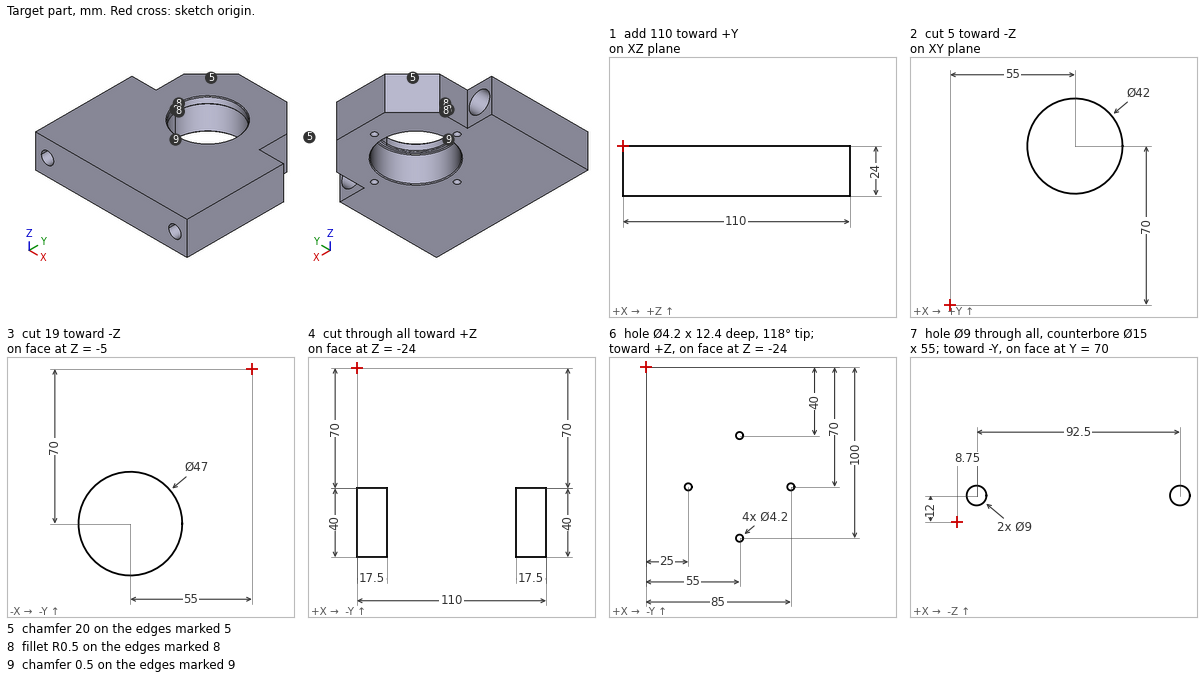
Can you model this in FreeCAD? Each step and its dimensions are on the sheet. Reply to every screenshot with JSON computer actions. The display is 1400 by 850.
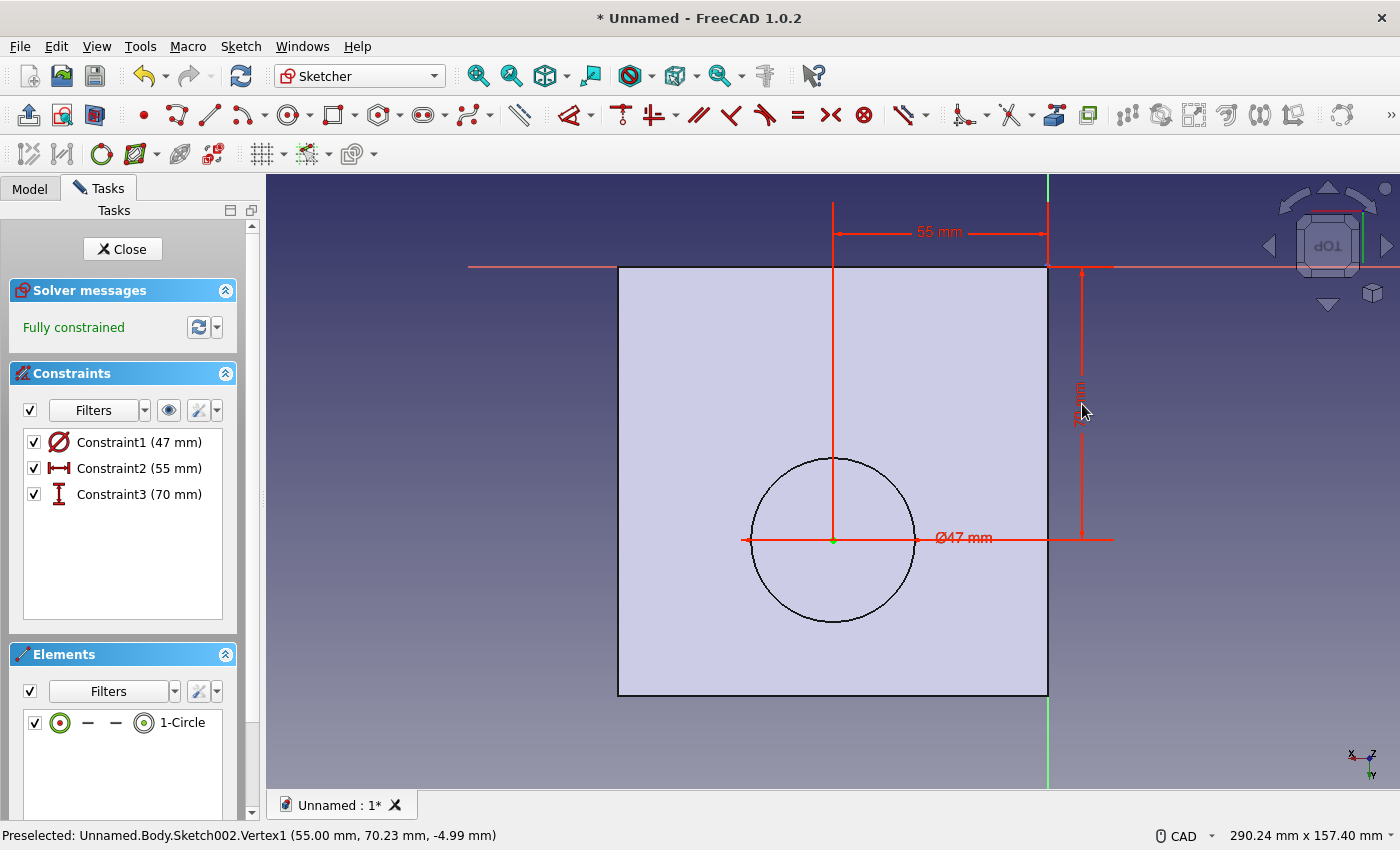
{"action": "left_click", "coordinate": [123, 249]}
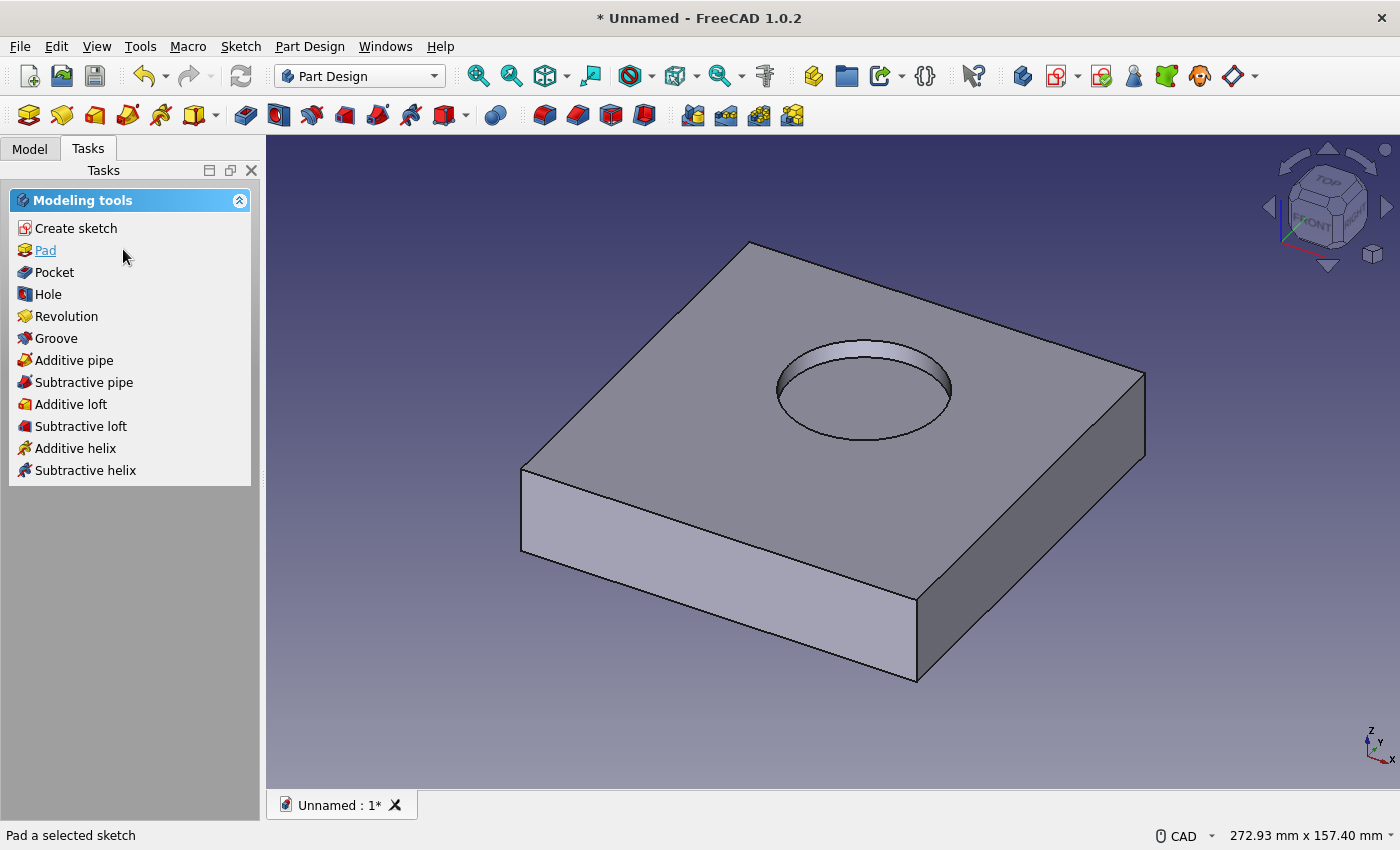
{"action": "left_click", "coordinate": [246, 116]}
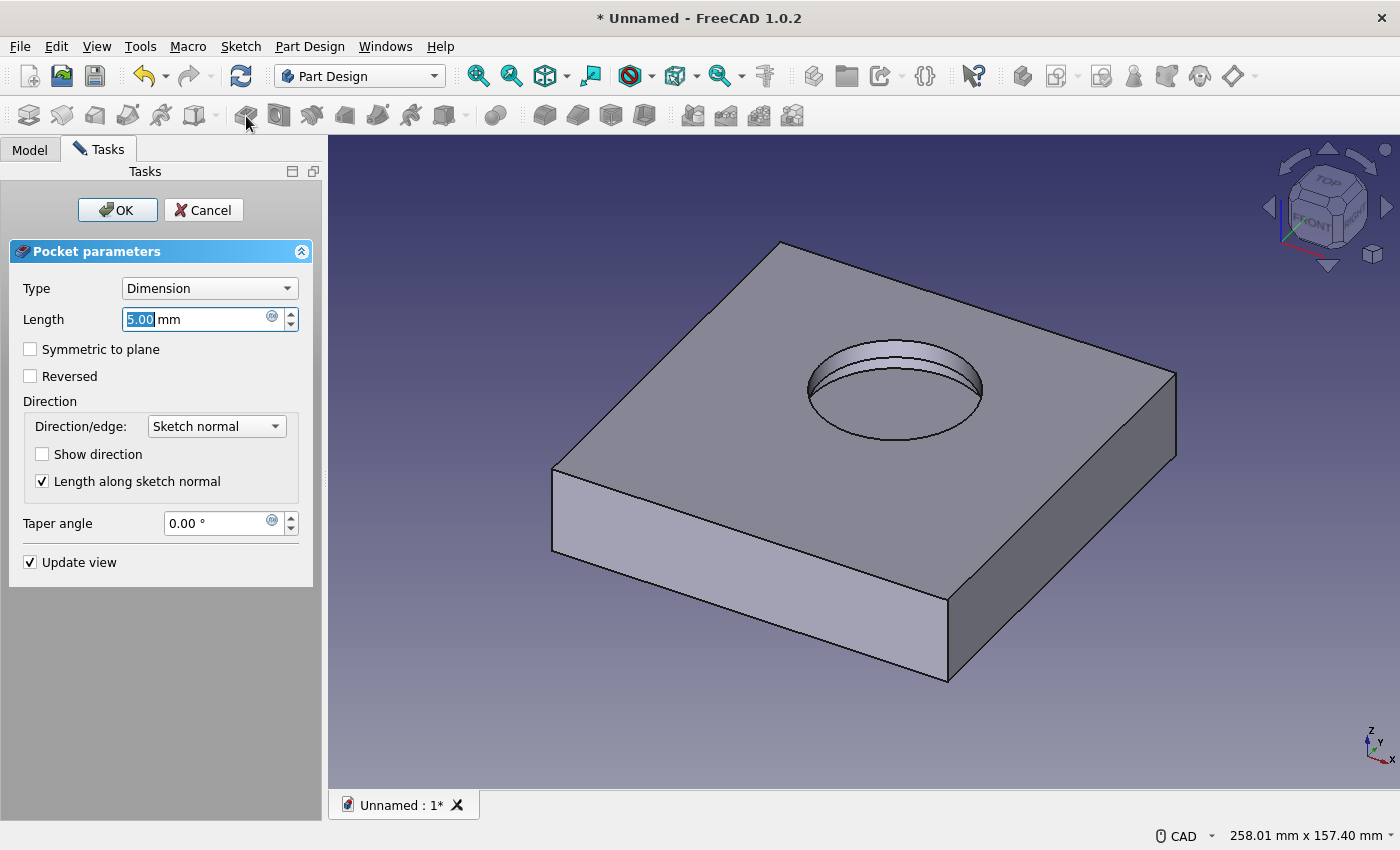
{"action": "type", "text": "19"}
{"action": "key", "text": "Tab"}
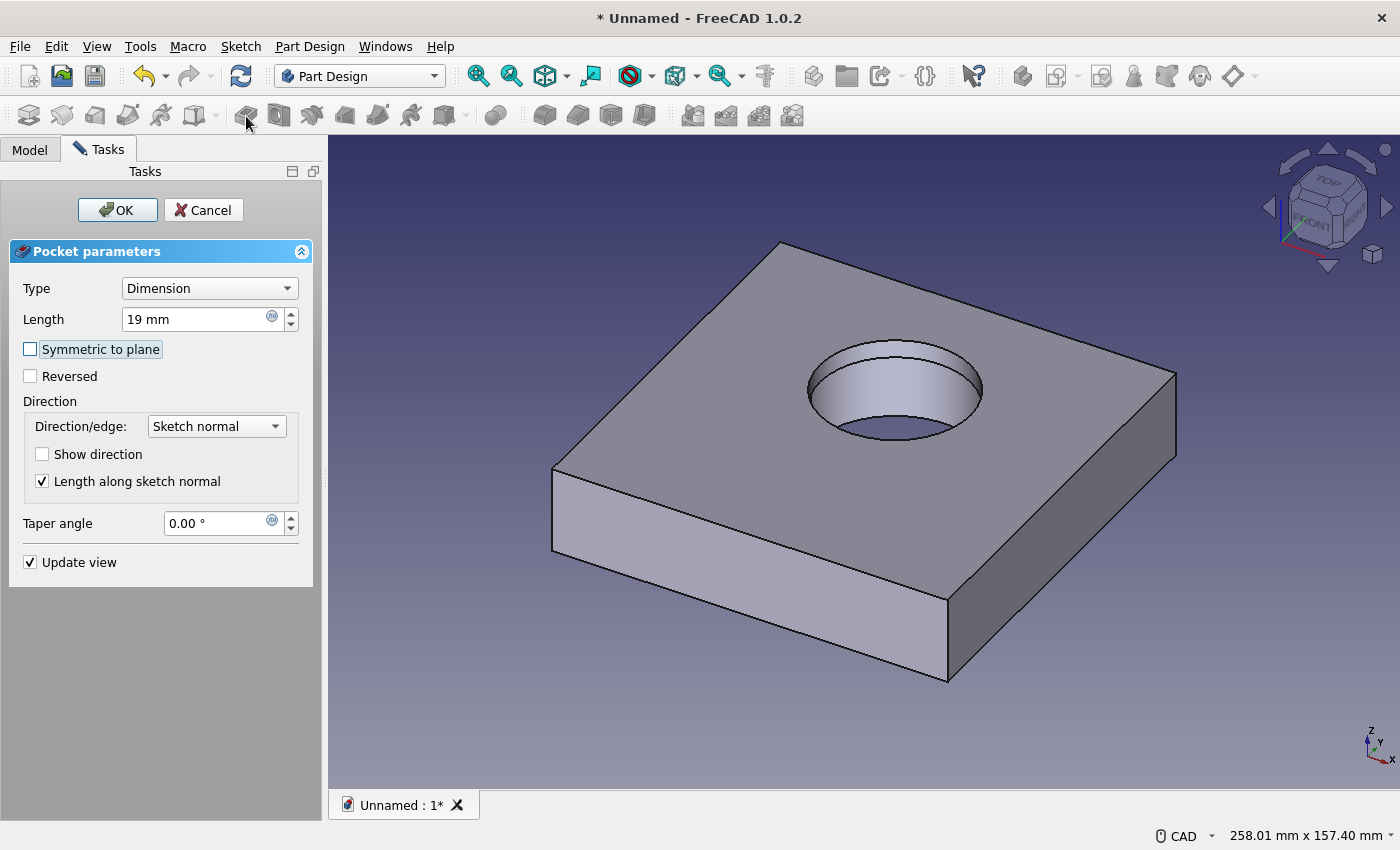
{"action": "left_click", "coordinate": [118, 210]}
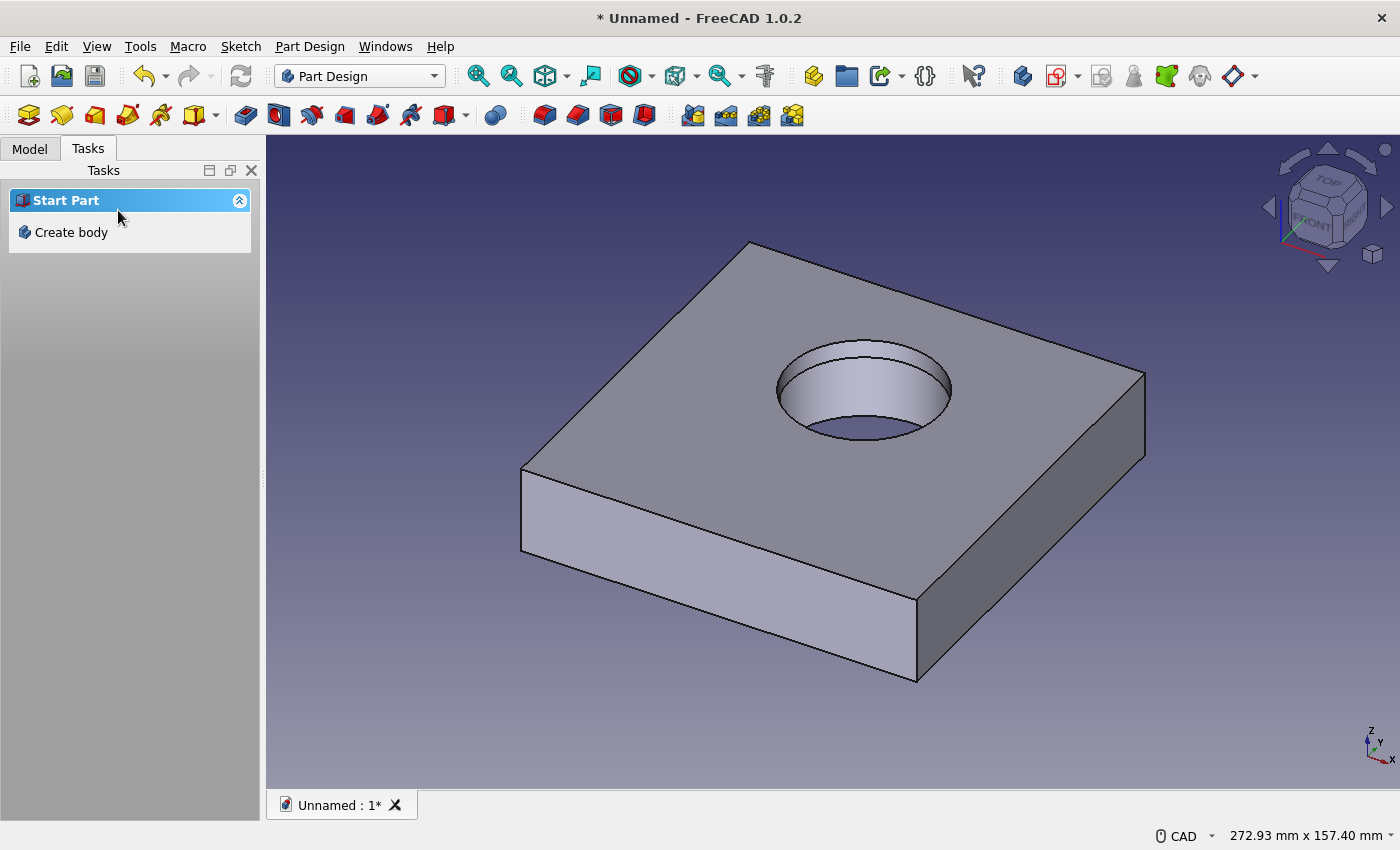
{"action": "key", "text": "5"}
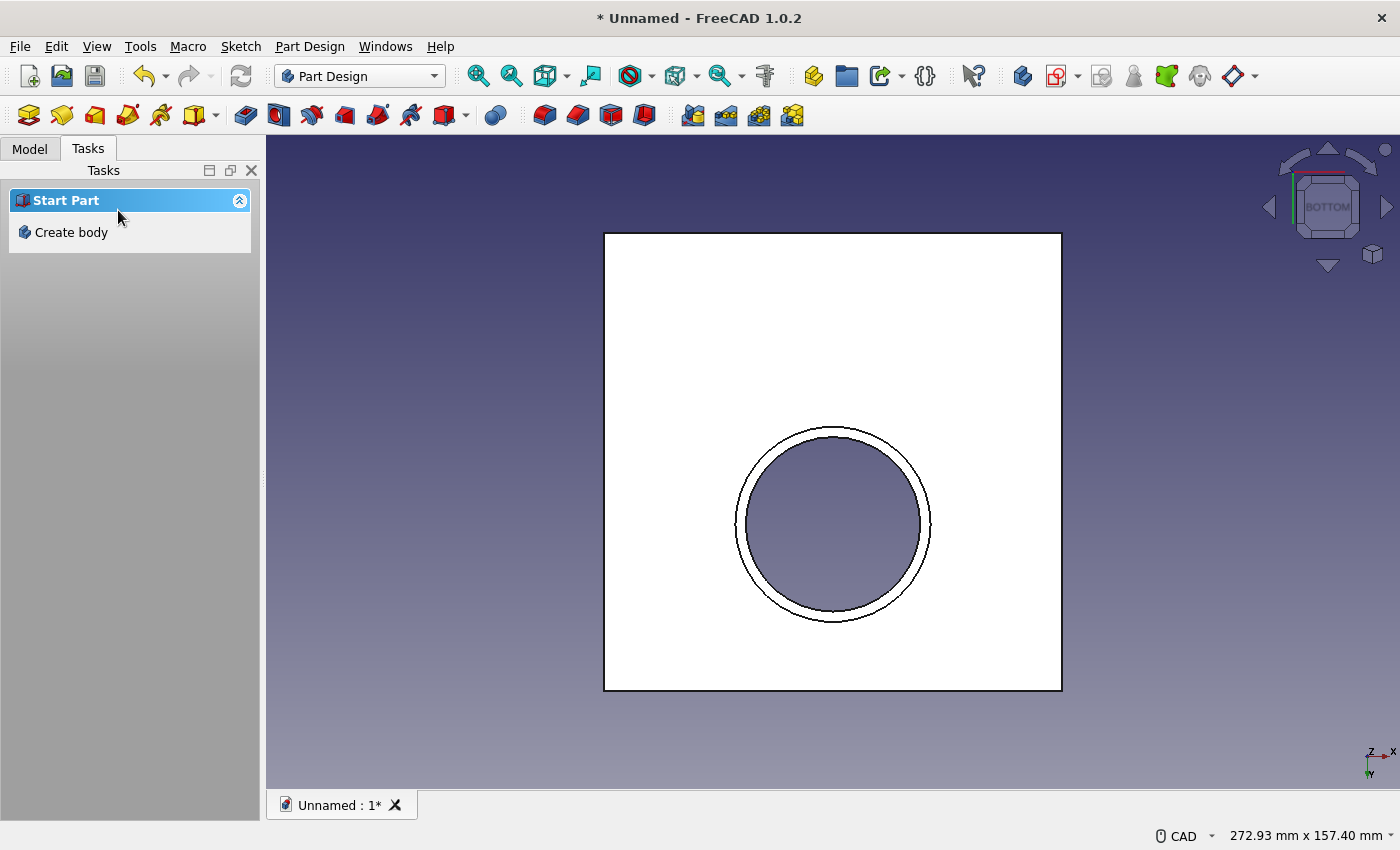
{"action": "left_click", "coordinate": [964, 330]}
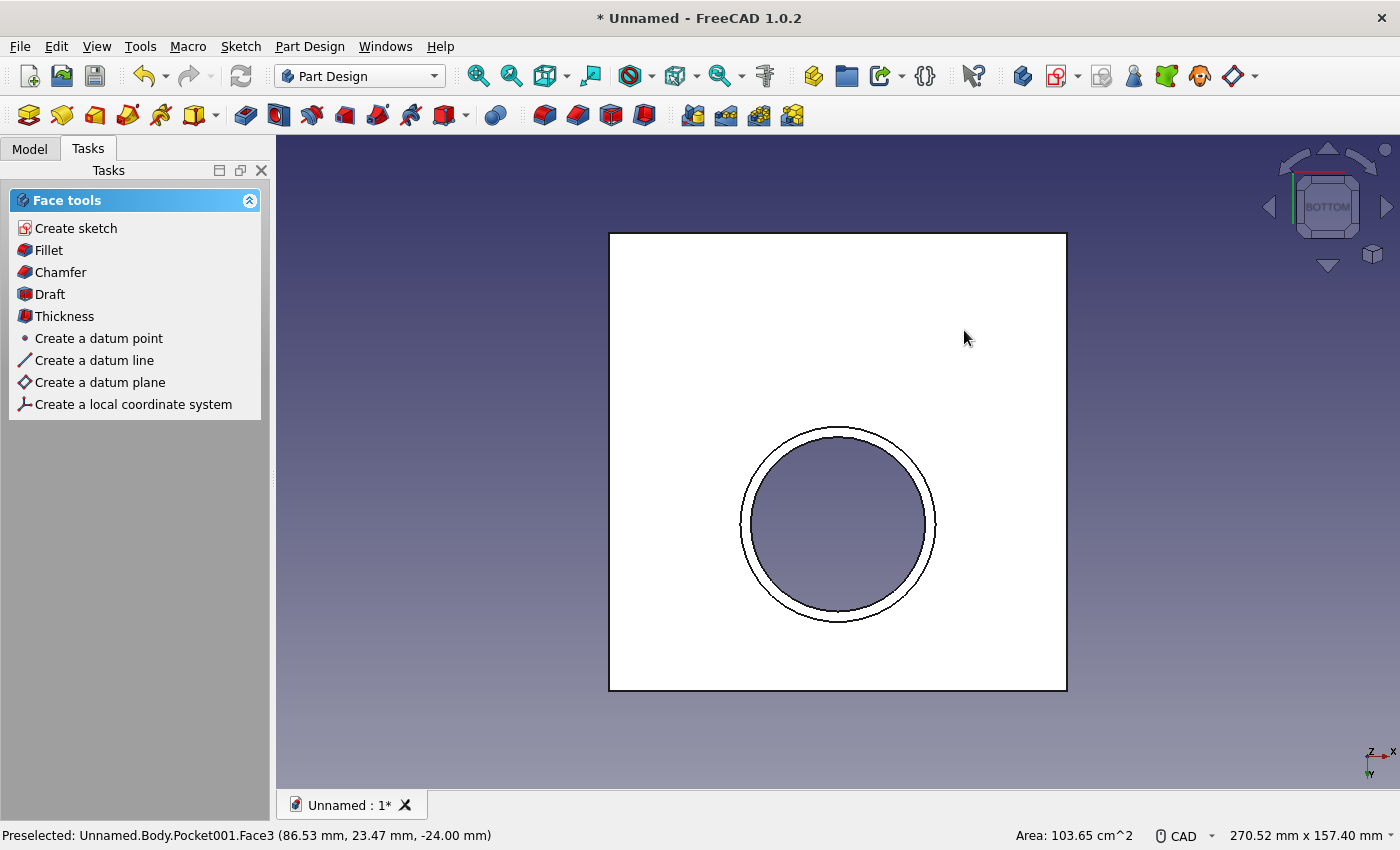
{"action": "left_click", "coordinate": [1056, 76]}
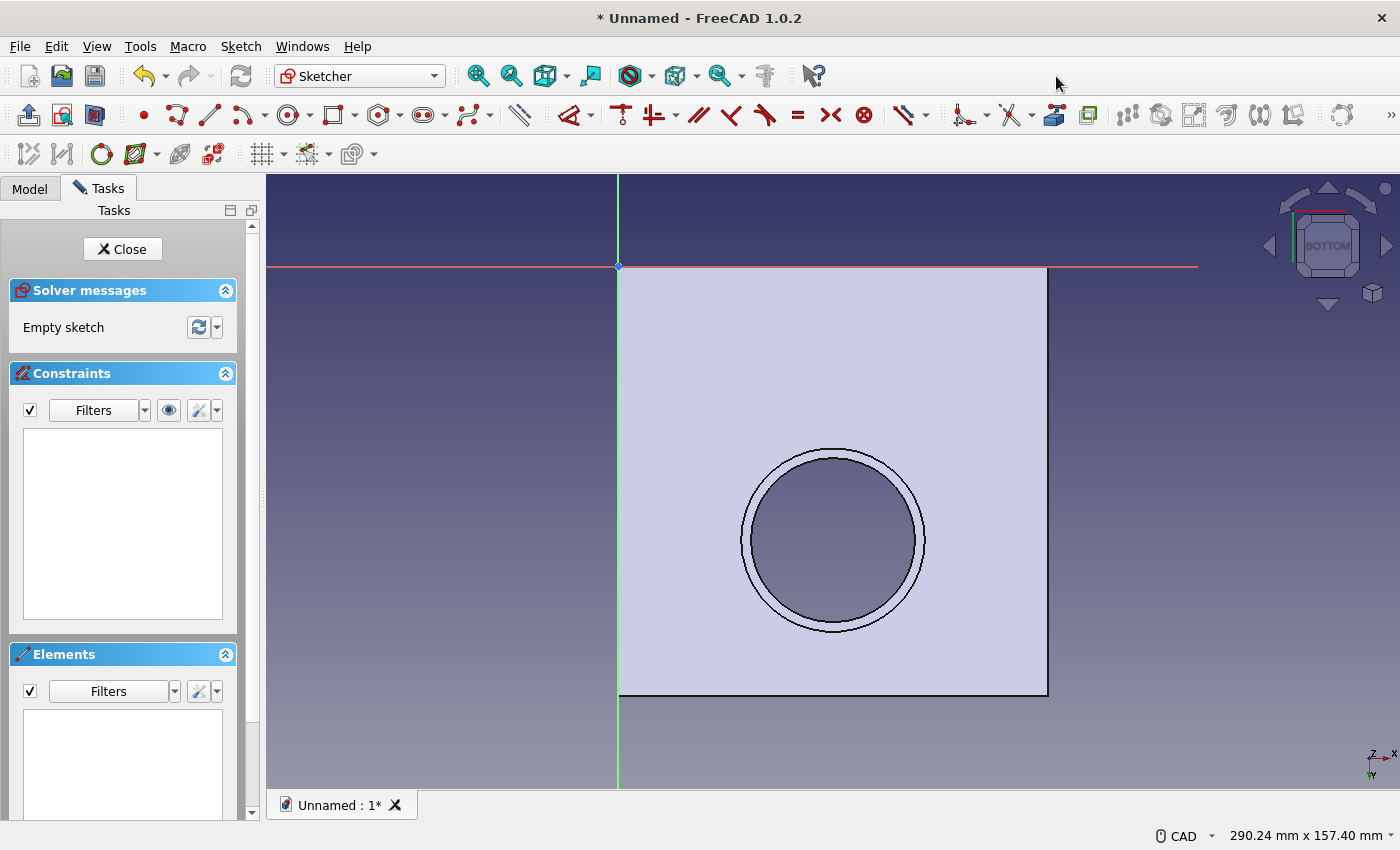
{"action": "left_click", "coordinate": [332, 116]}